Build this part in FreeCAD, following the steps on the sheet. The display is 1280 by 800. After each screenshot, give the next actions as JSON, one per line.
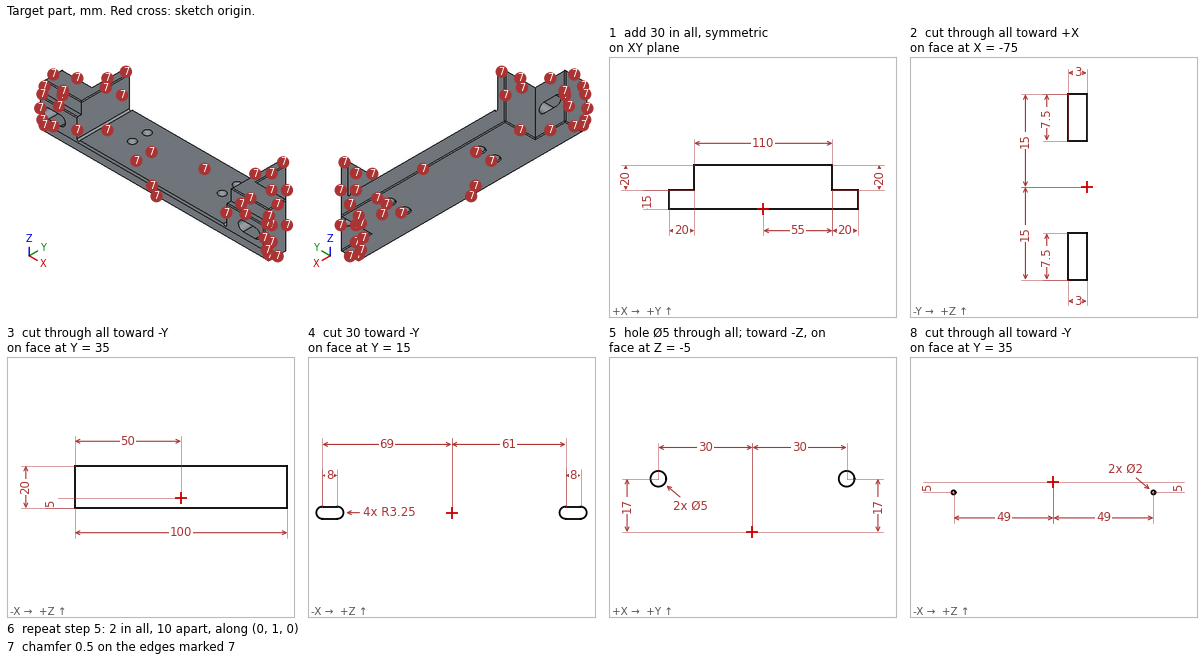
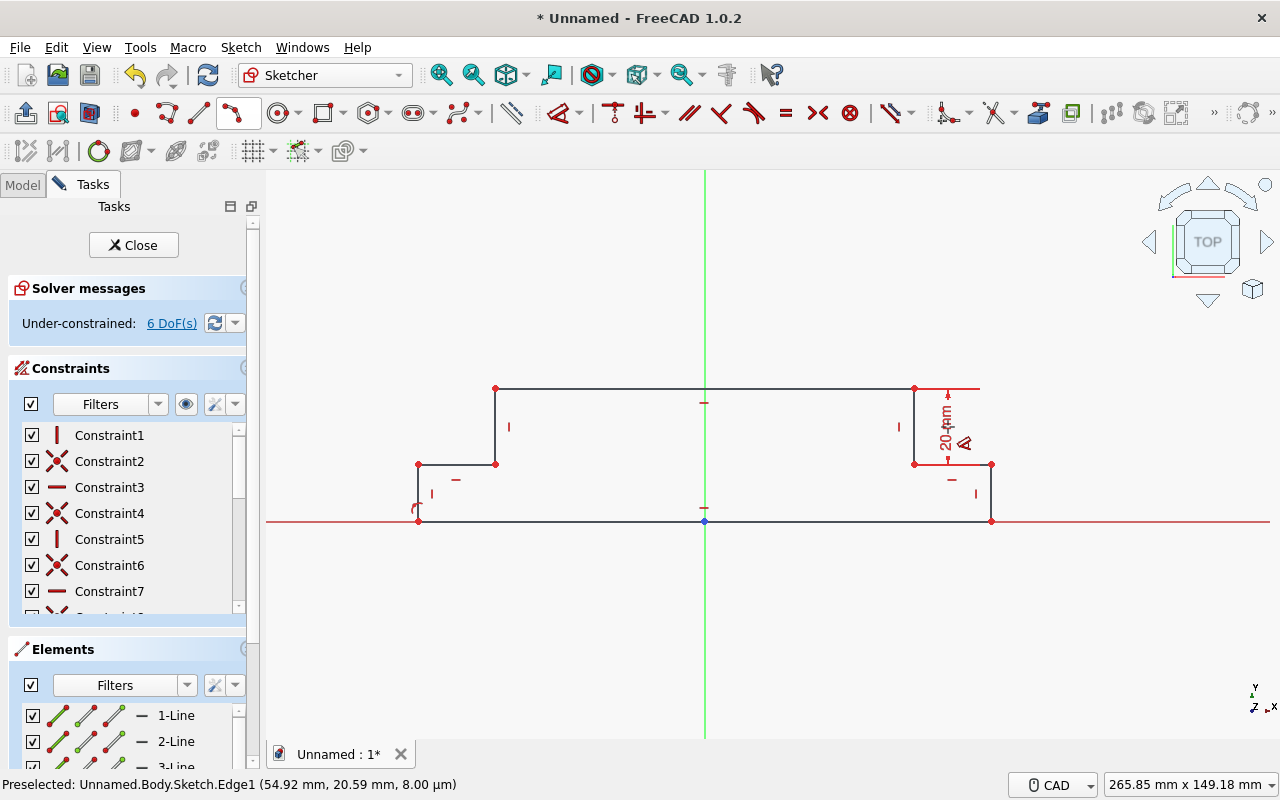
{"action": "left_click", "coordinate": [495, 412]}
{"action": "left_click", "coordinate": [461, 427]}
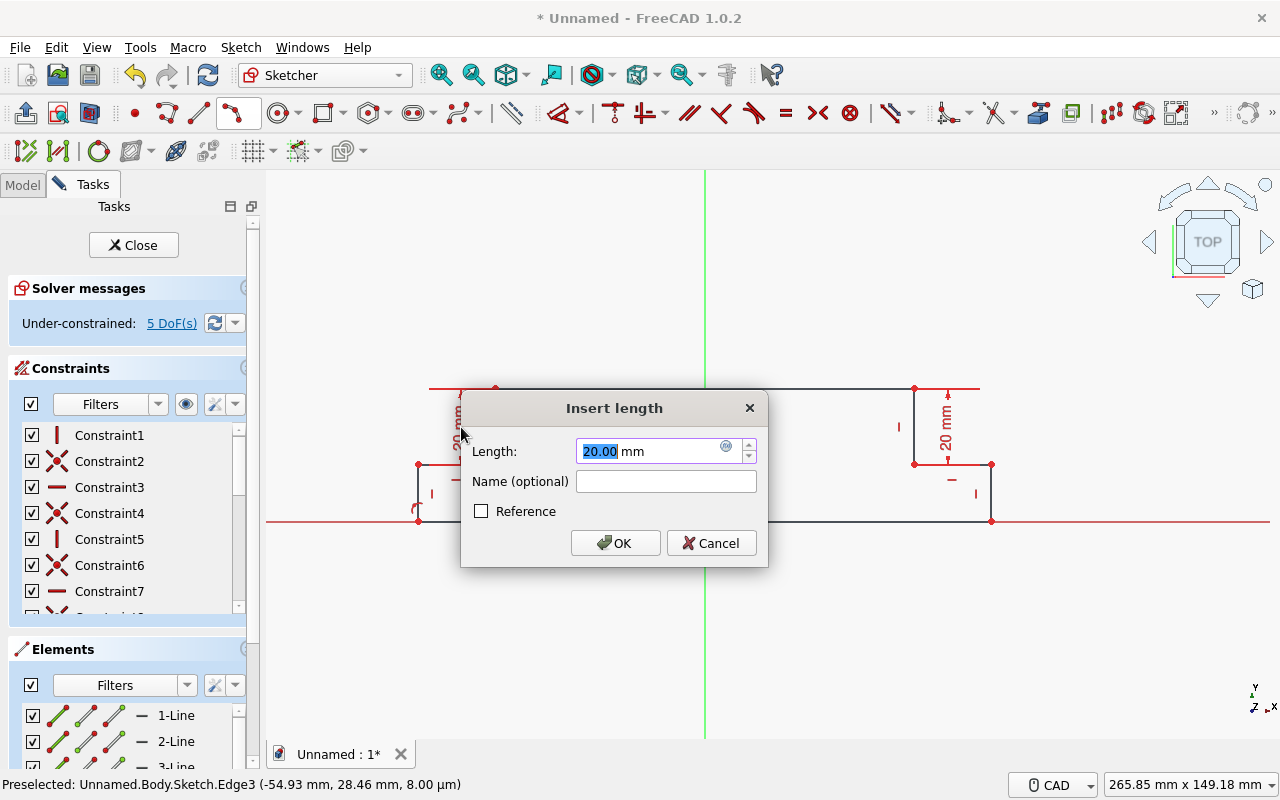
{"action": "type", "text": "20"}
{"action": "key", "text": "Return"}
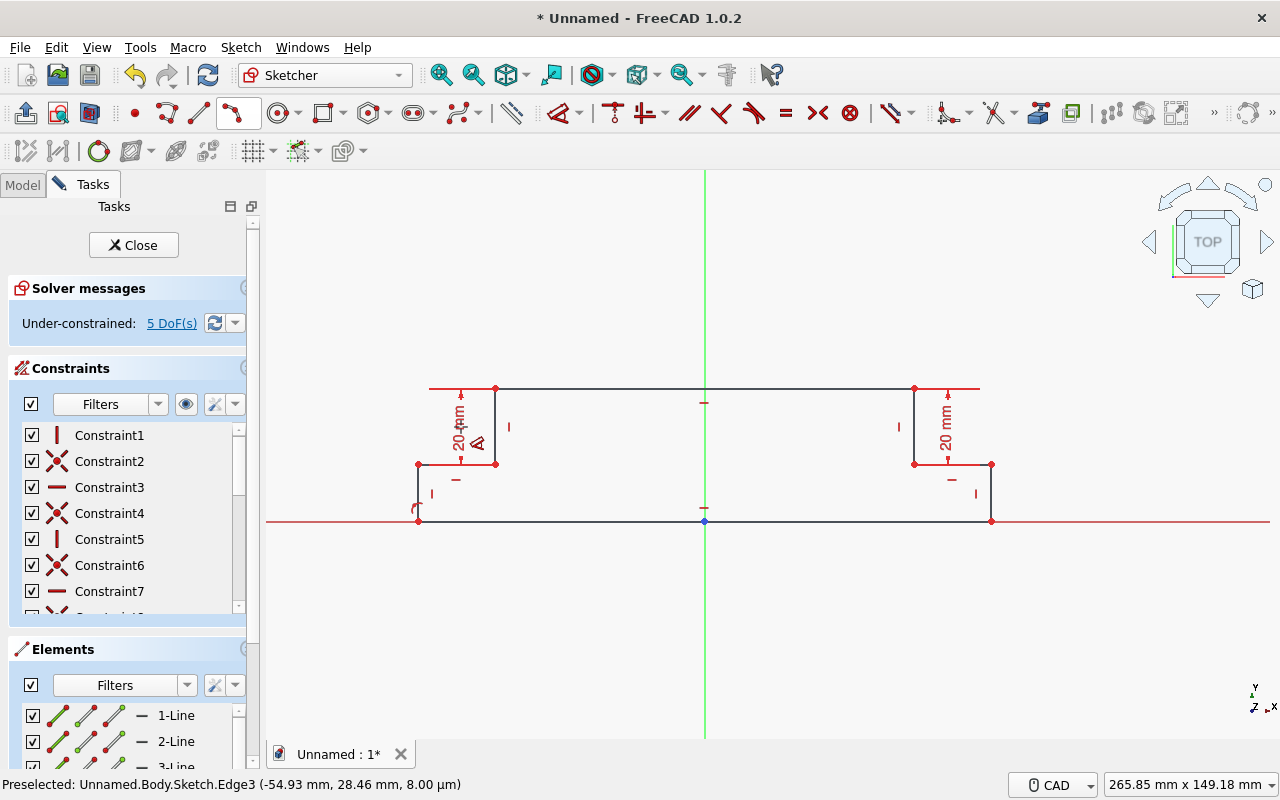
{"action": "left_click", "coordinate": [472, 465]}
{"action": "left_click", "coordinate": [456, 499]}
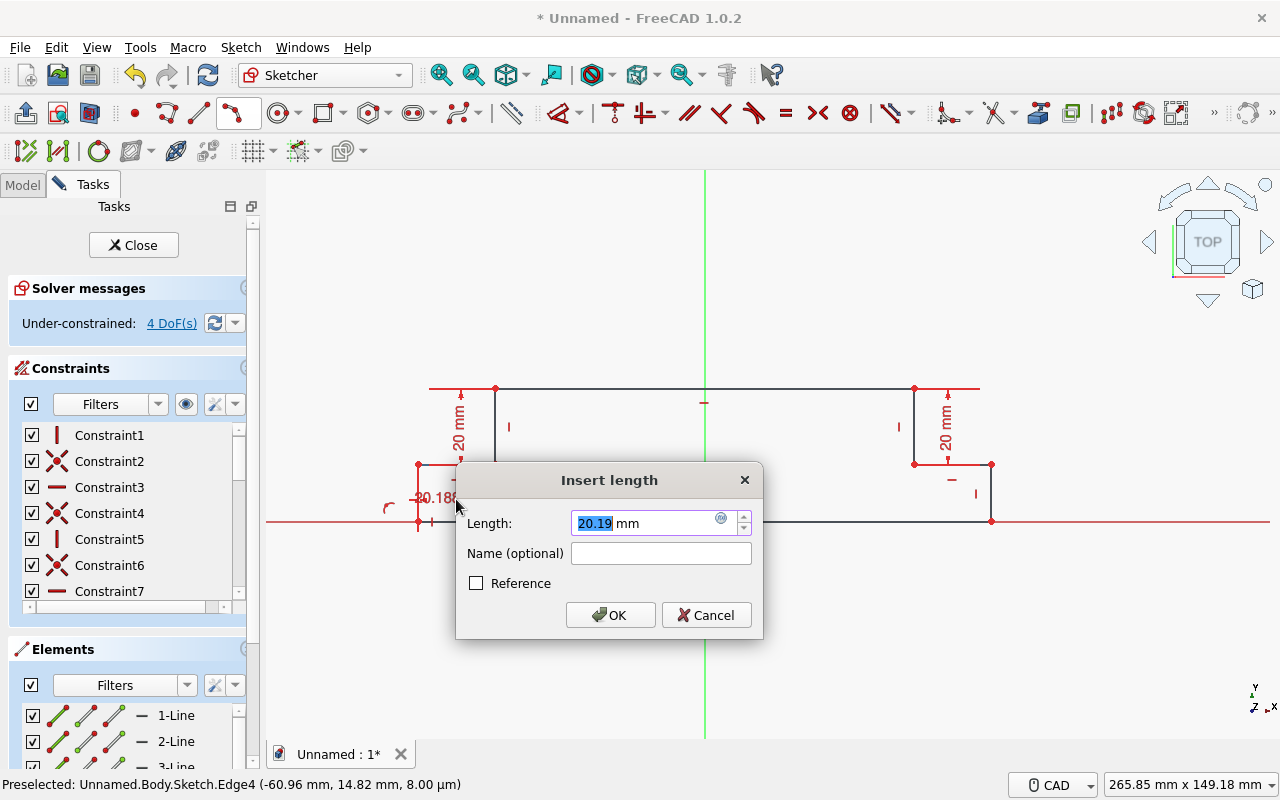
{"action": "type", "text": "20"}
{"action": "key", "text": "Return"}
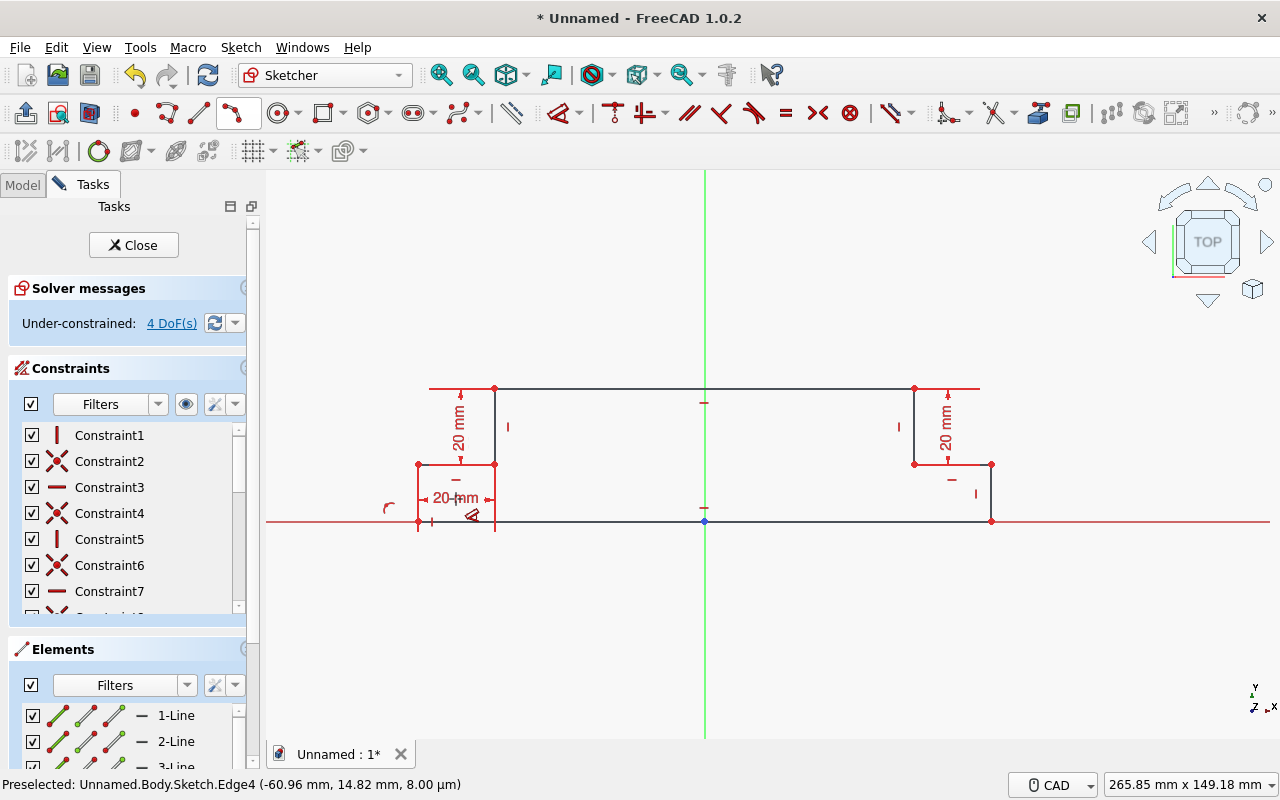
{"action": "left_click", "coordinate": [418, 482]}
{"action": "left_click", "coordinate": [384, 493]}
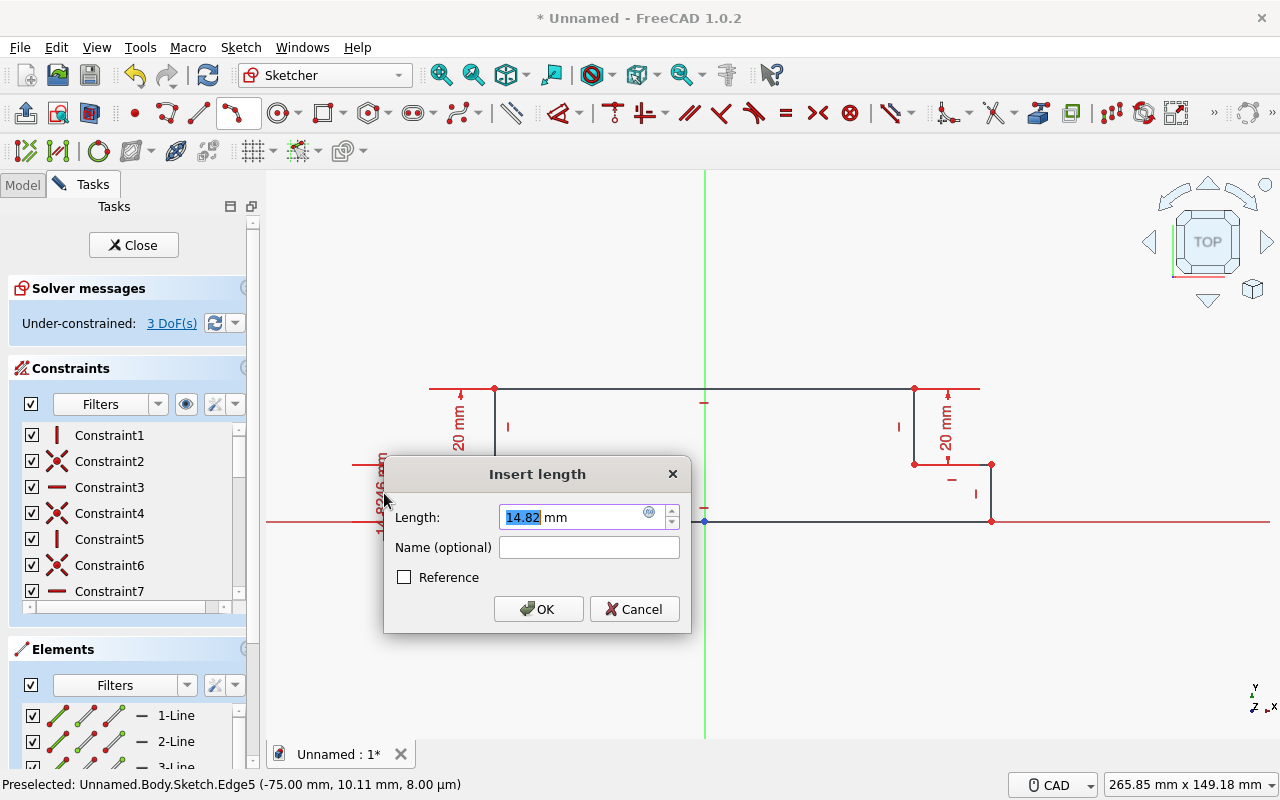
{"action": "type", "text": "15"}
{"action": "key", "text": "Return"}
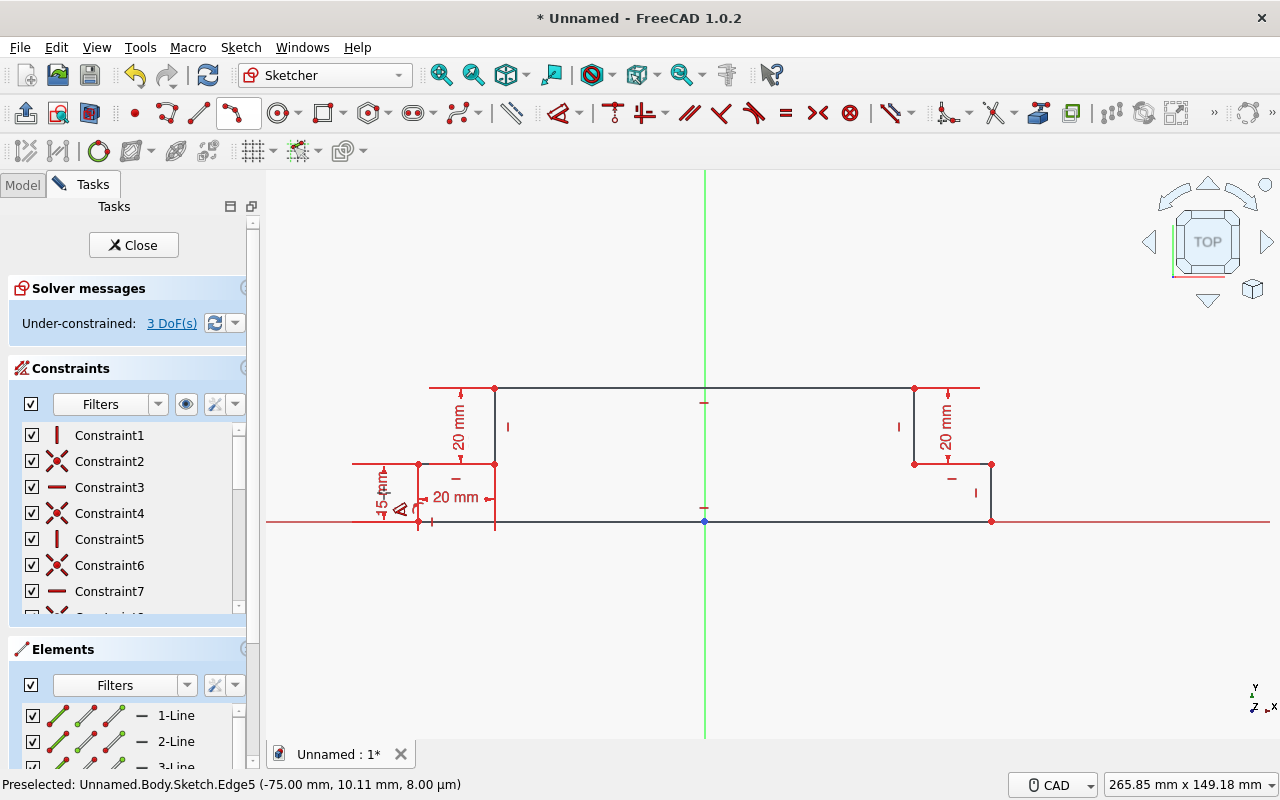
{"action": "left_click", "coordinate": [968, 464]}
{"action": "left_click", "coordinate": [952, 498]}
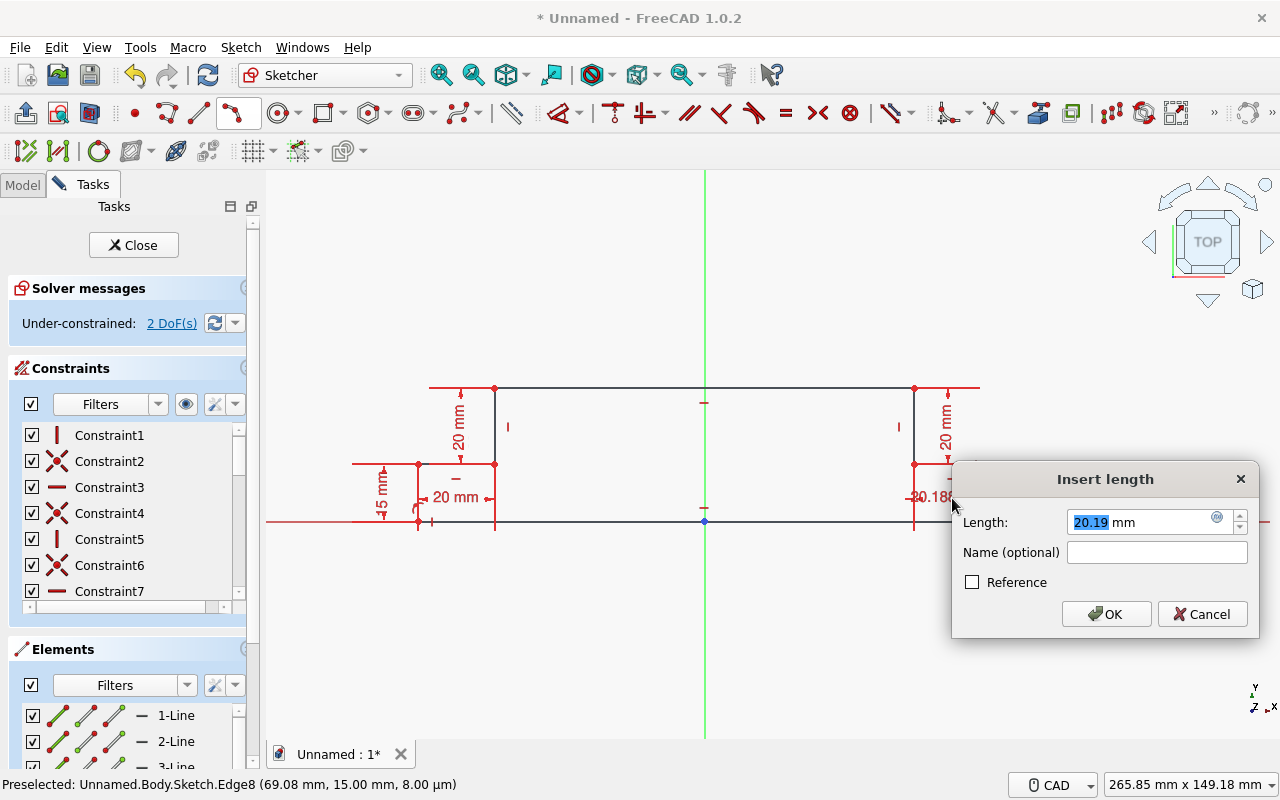
{"action": "type", "text": "20"}
{"action": "key", "text": "Return"}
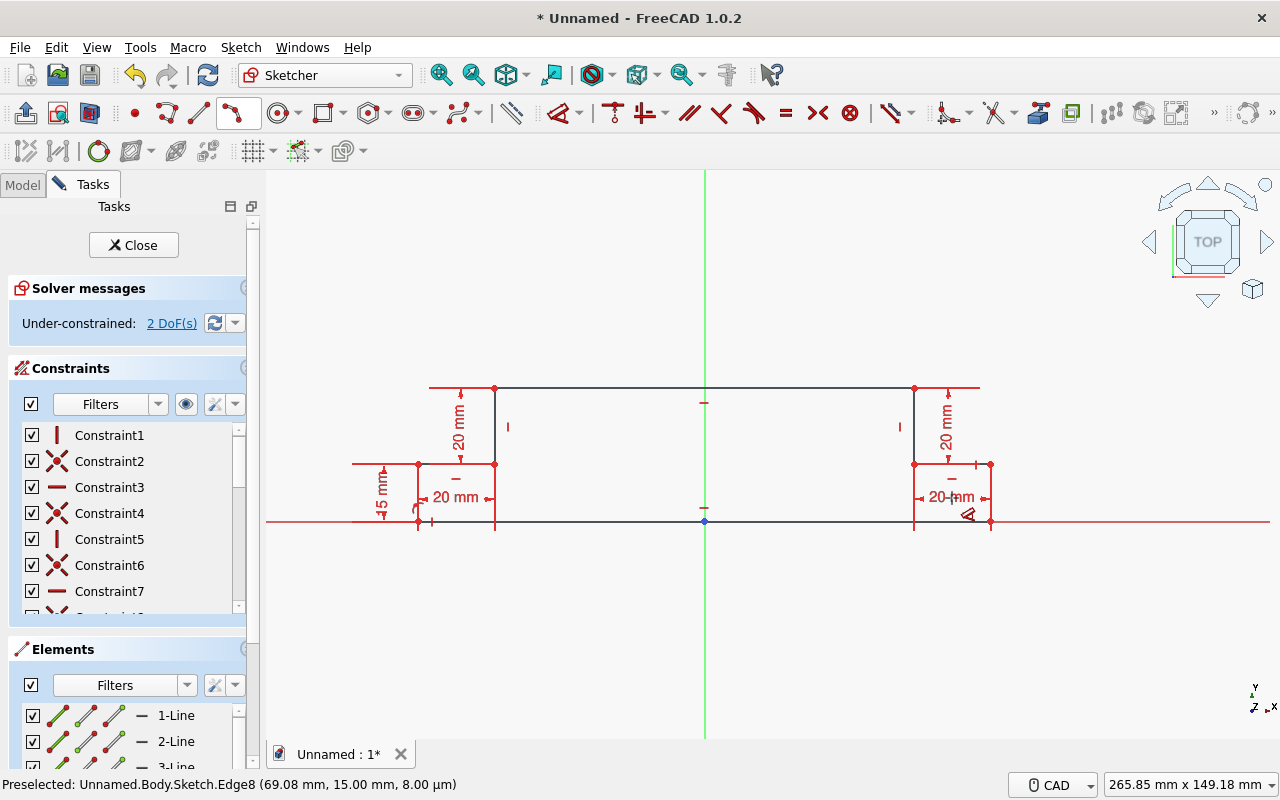
{"action": "left_click", "coordinate": [789, 388]}
{"action": "left_click", "coordinate": [608, 354]}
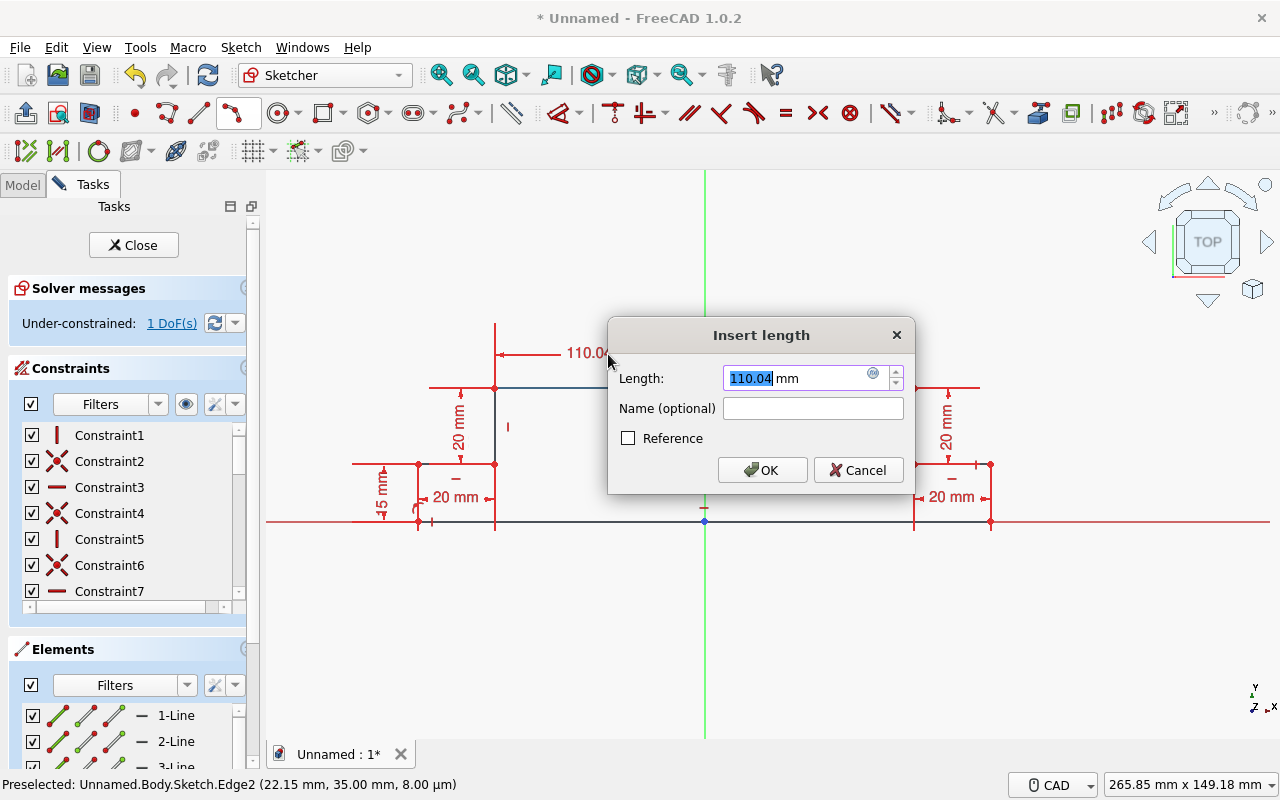
{"action": "type", "text": "110"}
{"action": "key", "text": "Return"}